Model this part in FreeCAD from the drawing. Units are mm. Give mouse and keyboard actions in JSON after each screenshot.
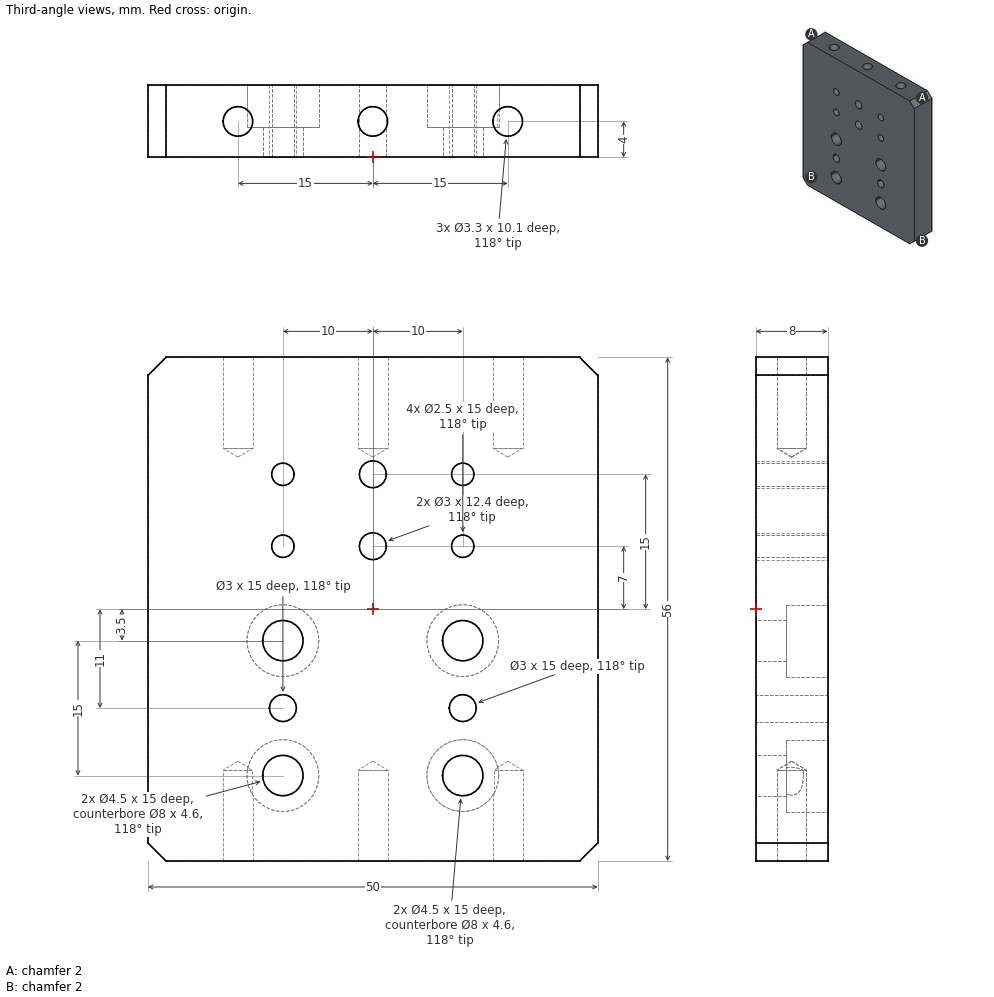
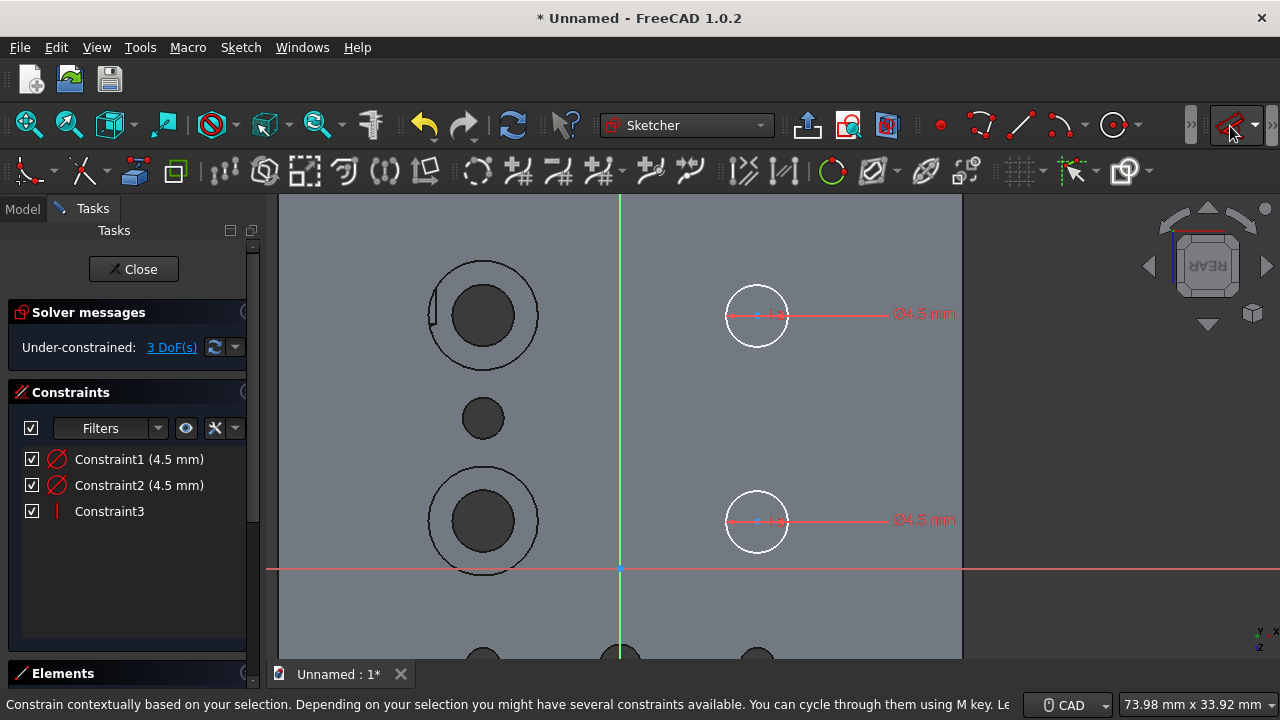
{"action": "left_click", "coordinate": [757, 316]}
{"action": "left_click", "coordinate": [689, 603]}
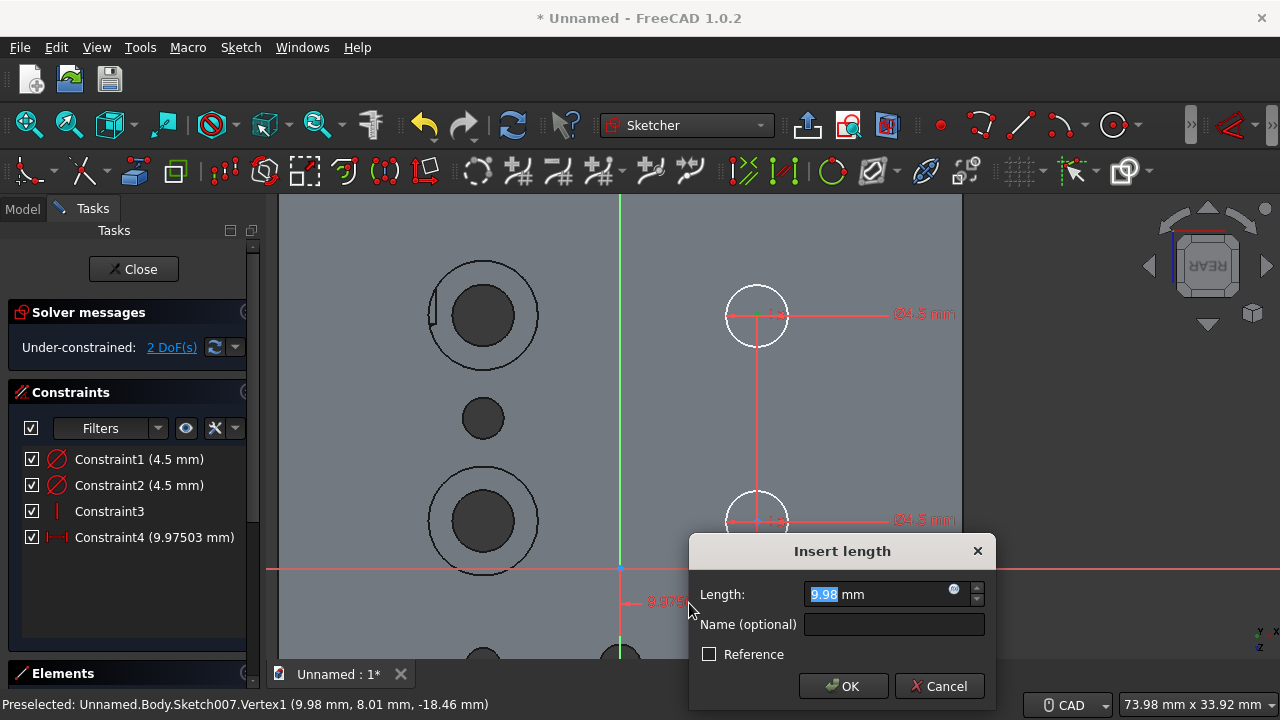
{"action": "type", "text": "10"}
{"action": "key", "text": "Return"}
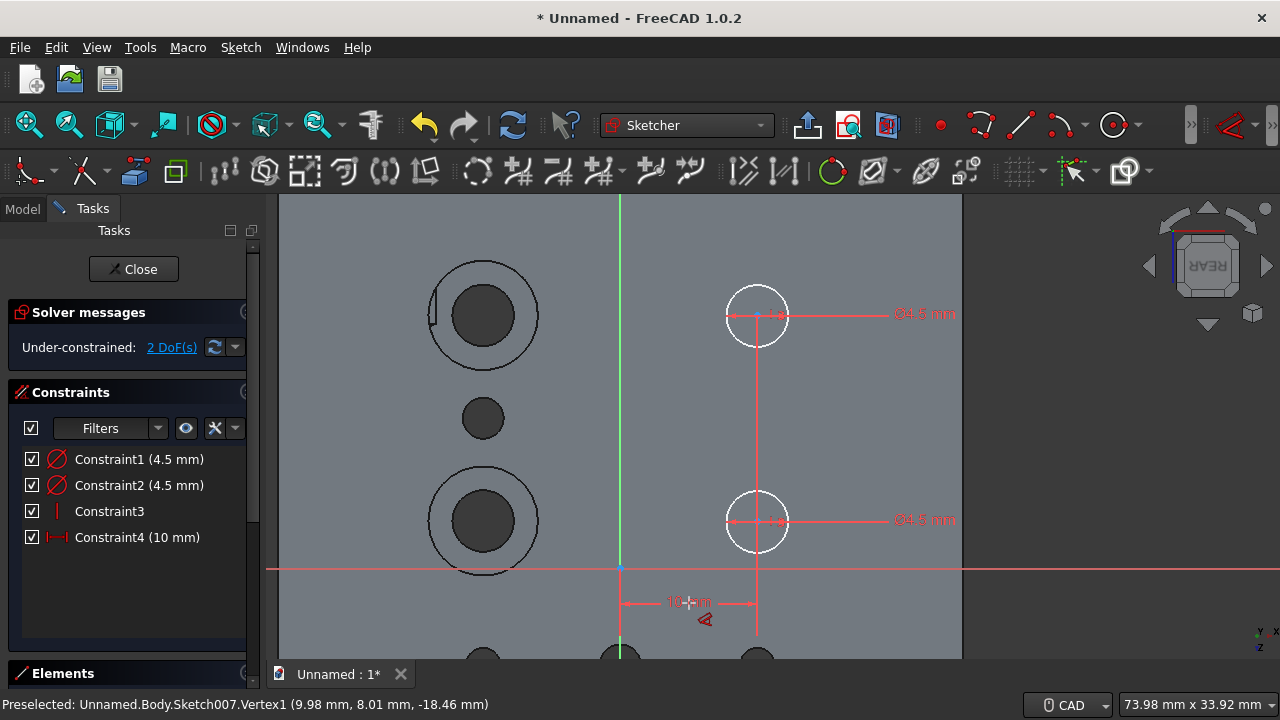
{"action": "left_click", "coordinate": [757, 522]}
{"action": "left_click", "coordinate": [586, 545]}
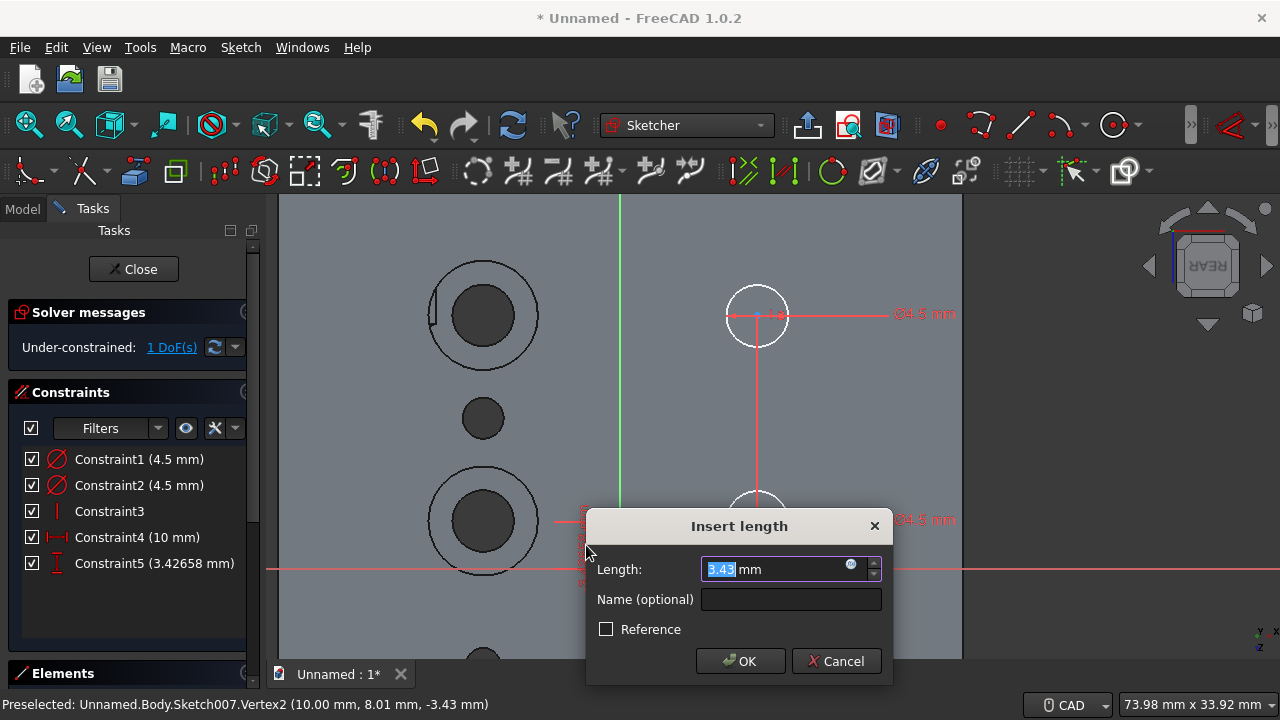
{"action": "type", "text": "3.5"}
{"action": "key", "text": "Return"}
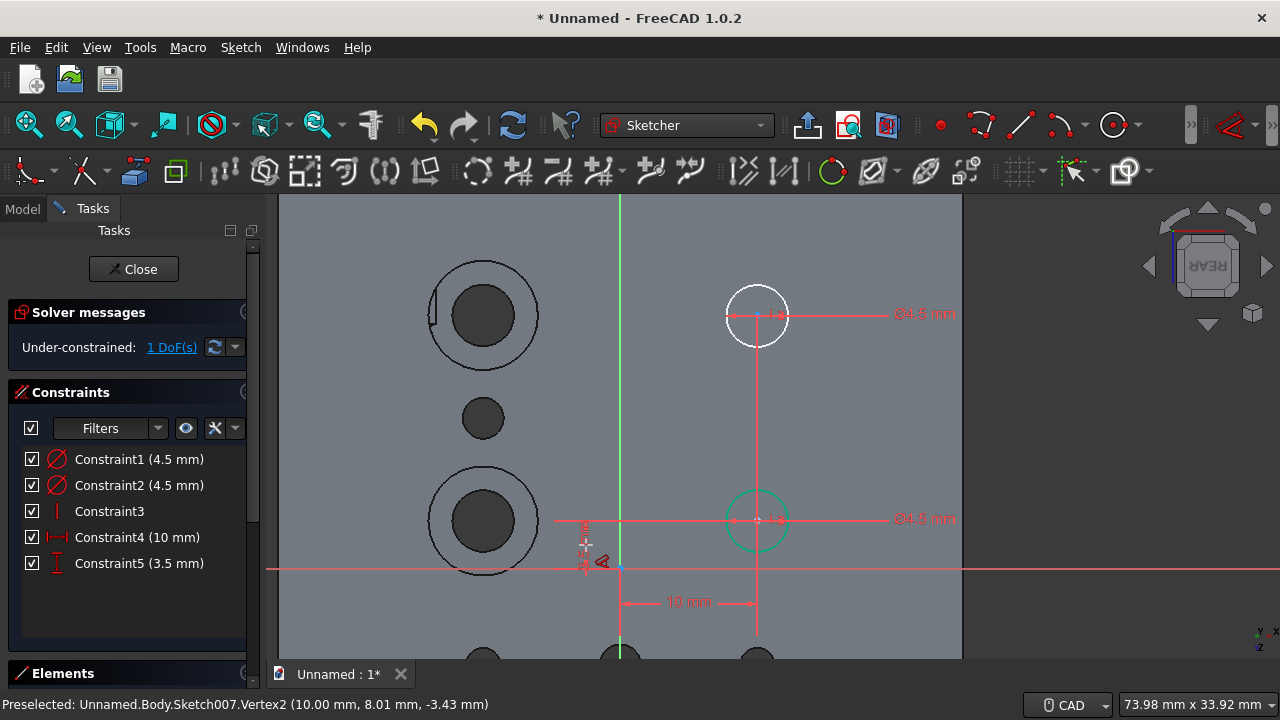
{"action": "left_click", "coordinate": [757, 316]}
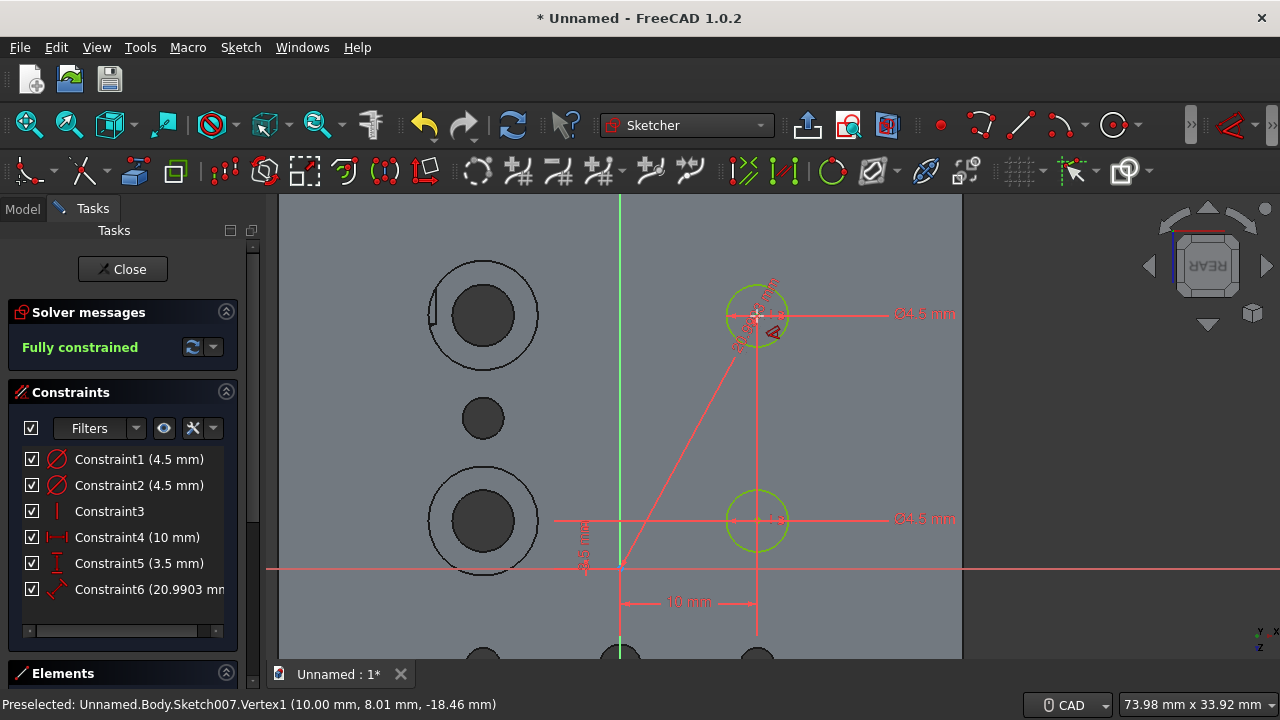
{"action": "left_click", "coordinate": [757, 521]}
{"action": "left_click", "coordinate": [791, 418]}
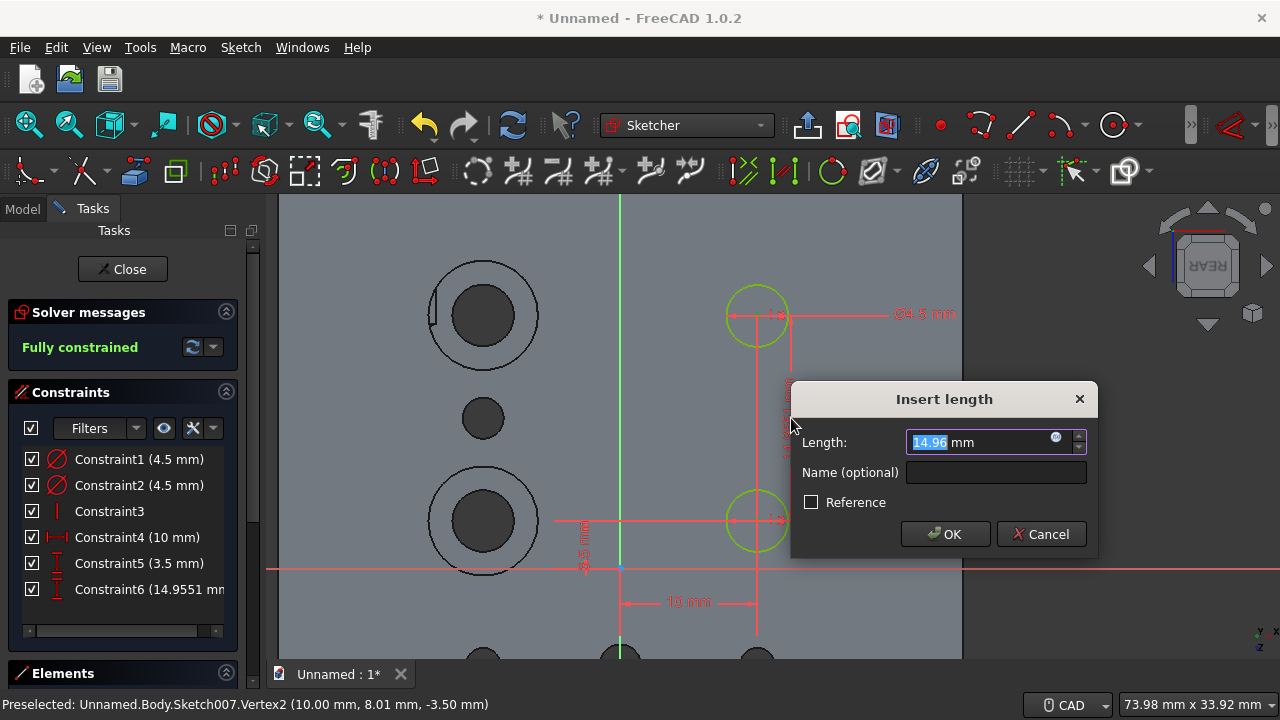
{"action": "type", "text": "15"}
{"action": "key", "text": "Return"}
{"action": "key", "text": "Escape"}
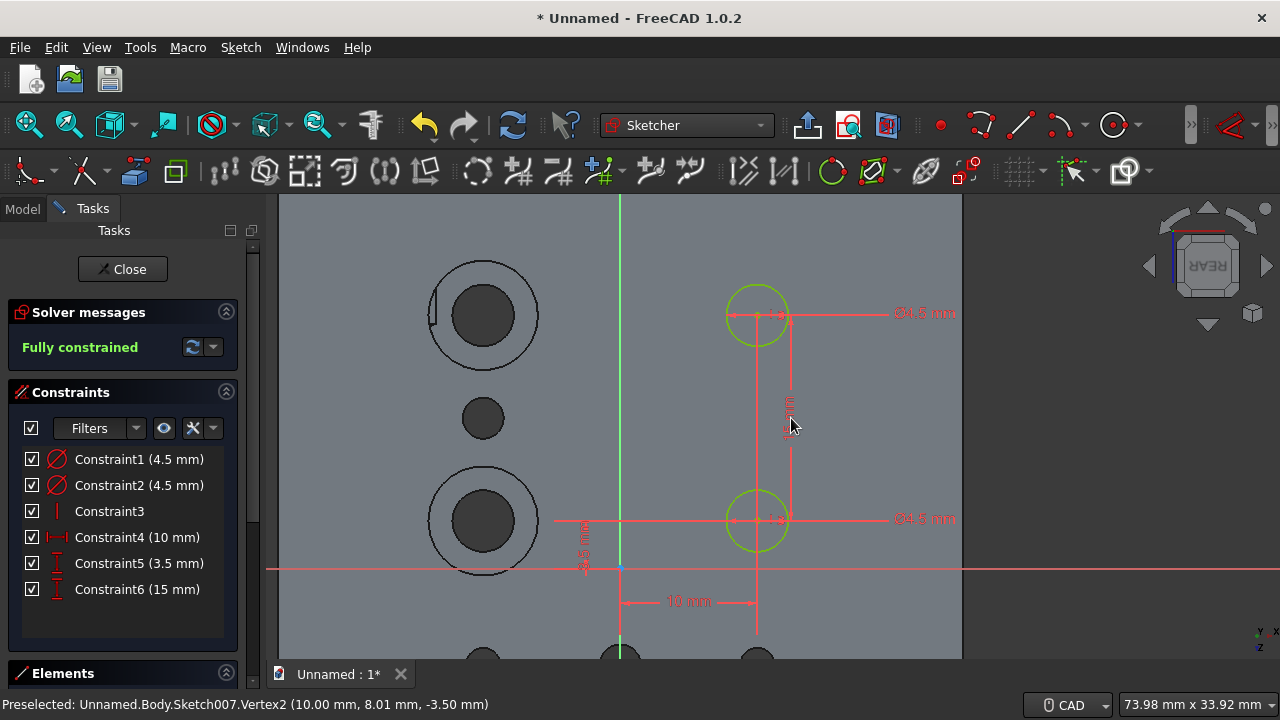
{"action": "left_click", "coordinate": [123, 269]}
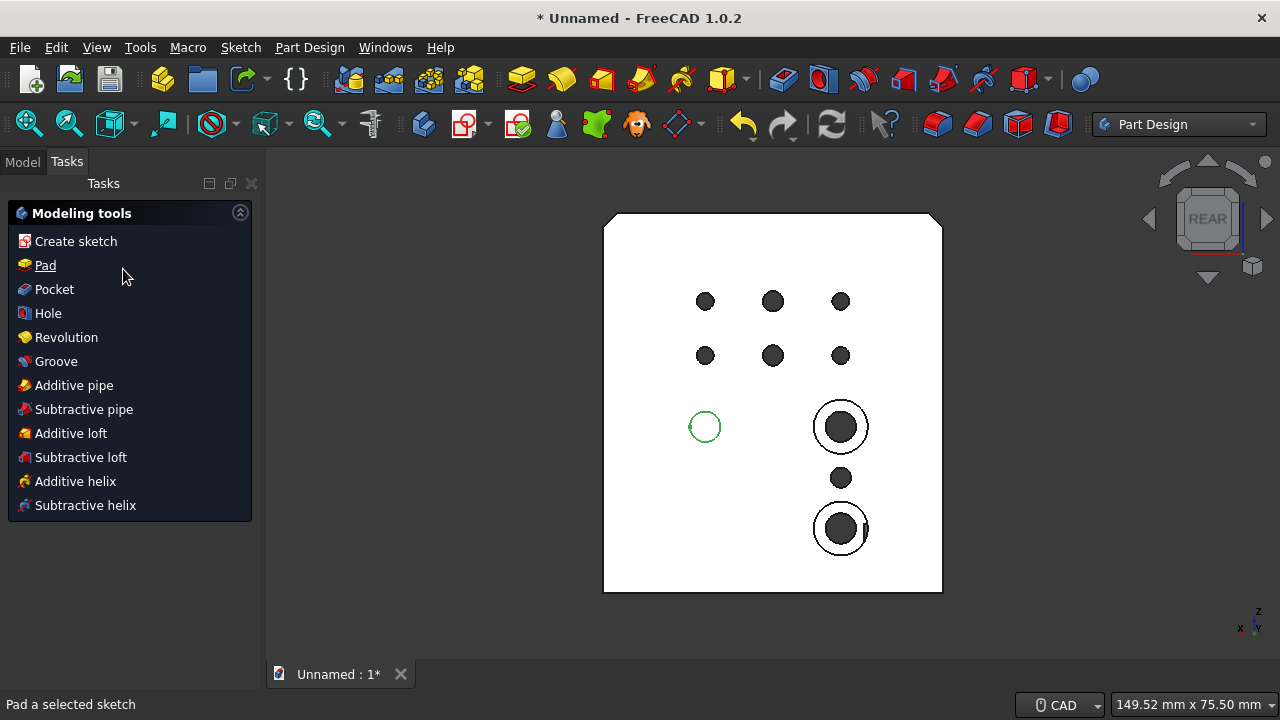
{"action": "left_click", "coordinate": [824, 80]}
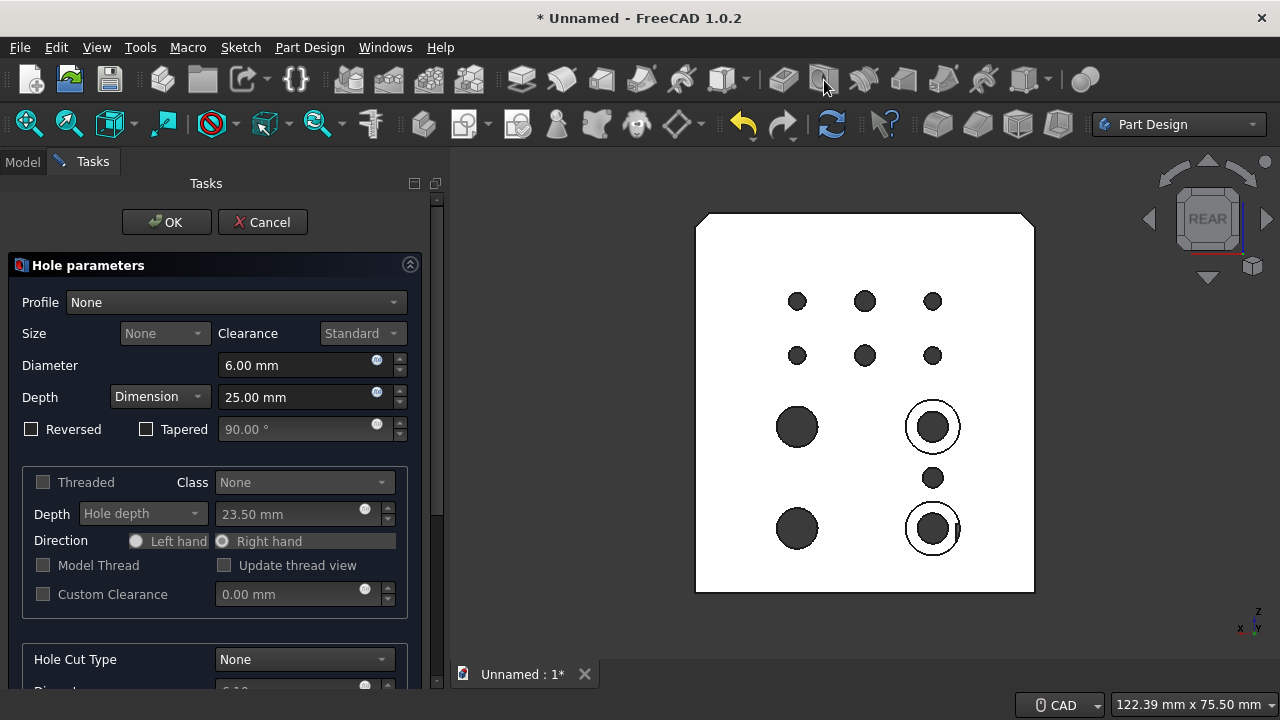
{"action": "triple_click", "coordinate": [305, 365]}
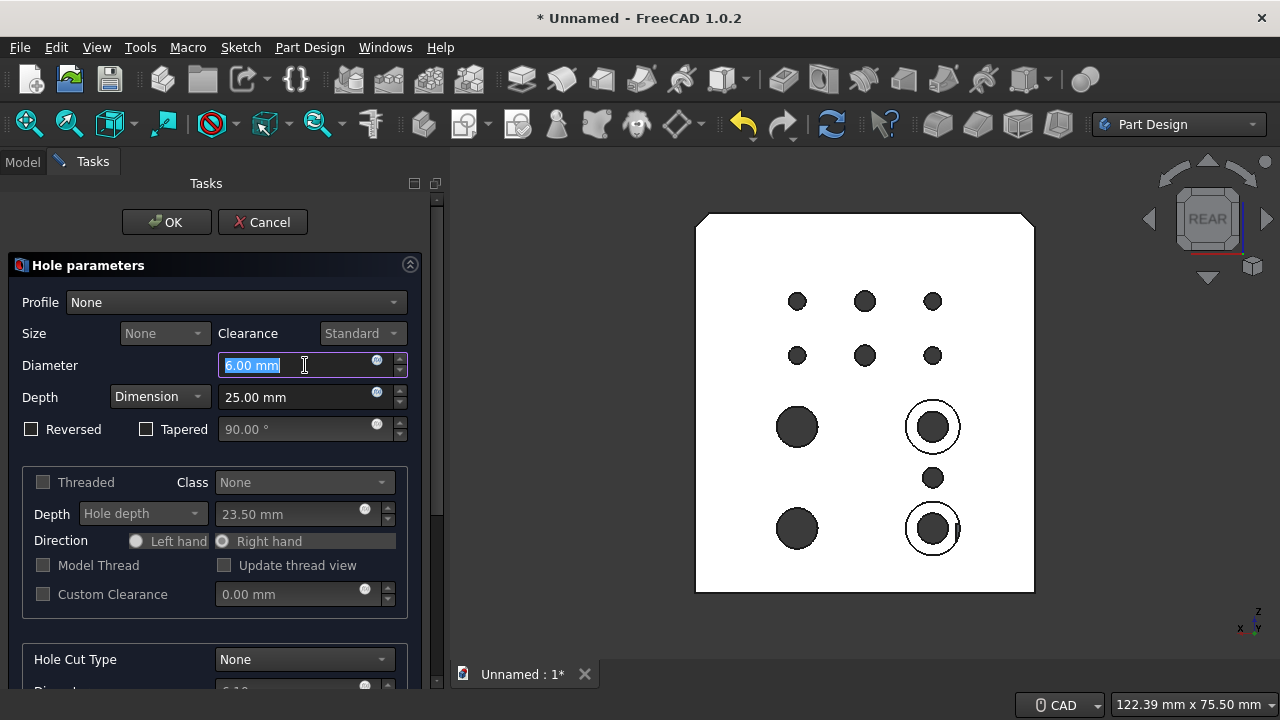
{"action": "type", "text": "4.5"}
{"action": "key", "text": "Tab"}